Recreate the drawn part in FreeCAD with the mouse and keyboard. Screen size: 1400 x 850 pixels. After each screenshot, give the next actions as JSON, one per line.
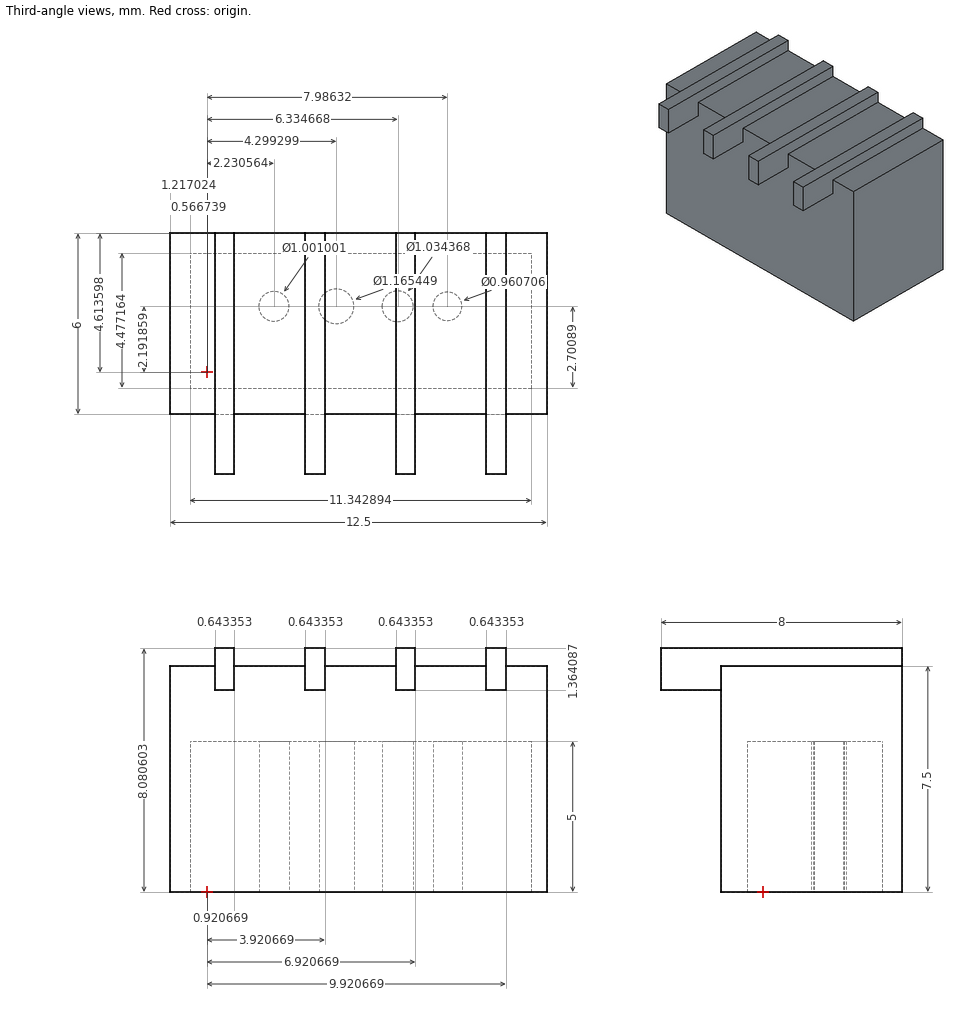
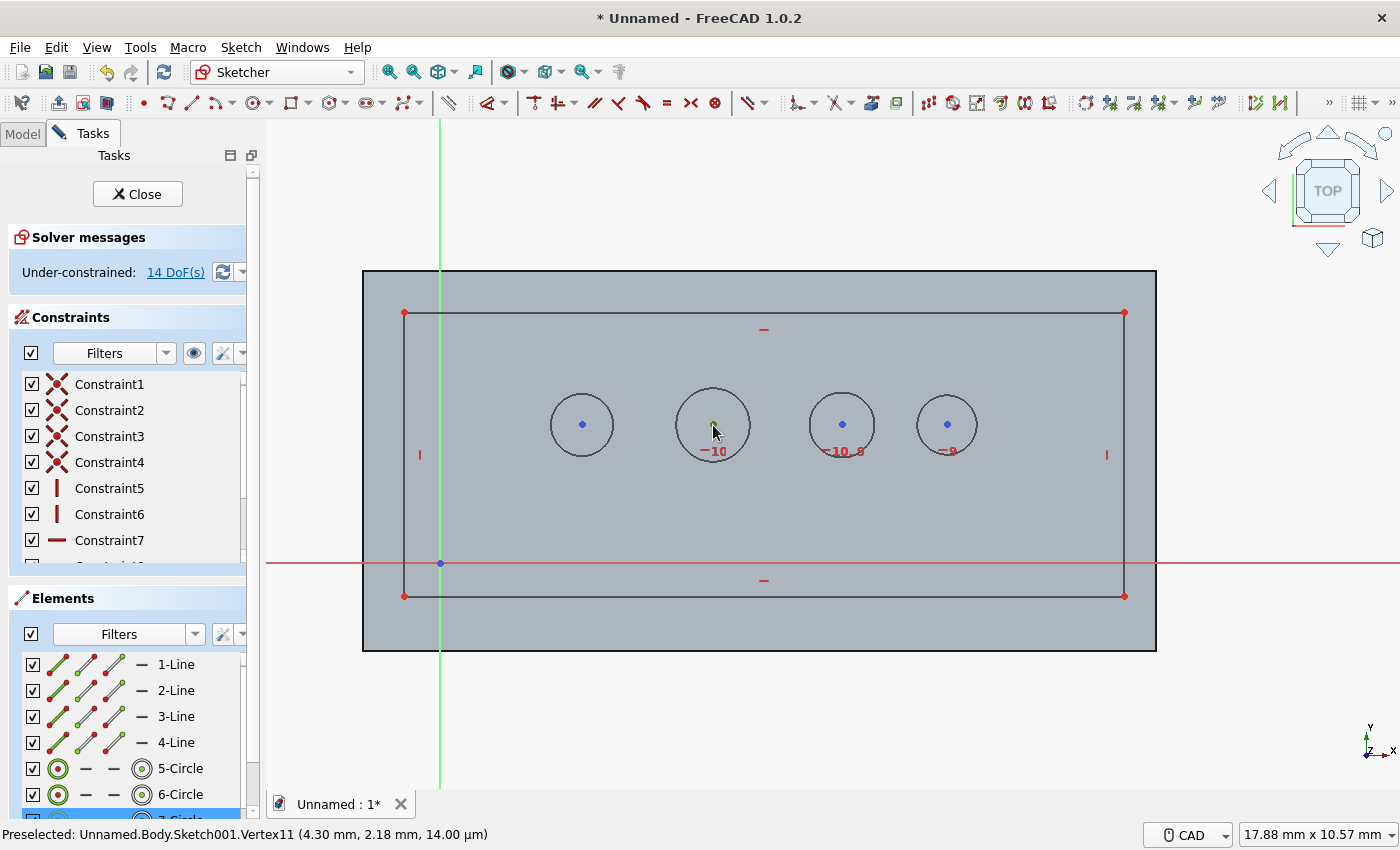
{"action": "left_click", "coordinate": [582, 425]}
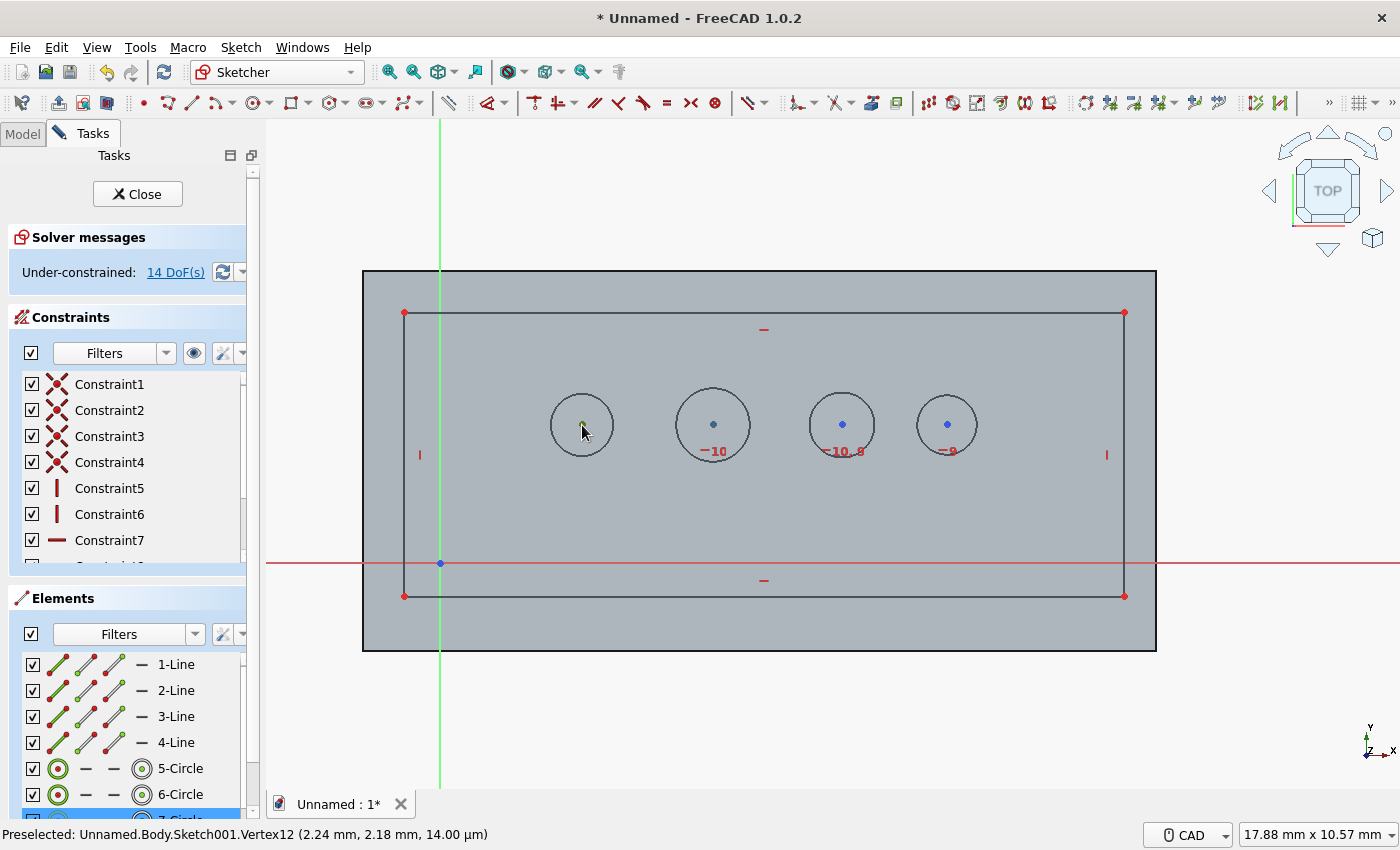
{"action": "key", "text": "h"}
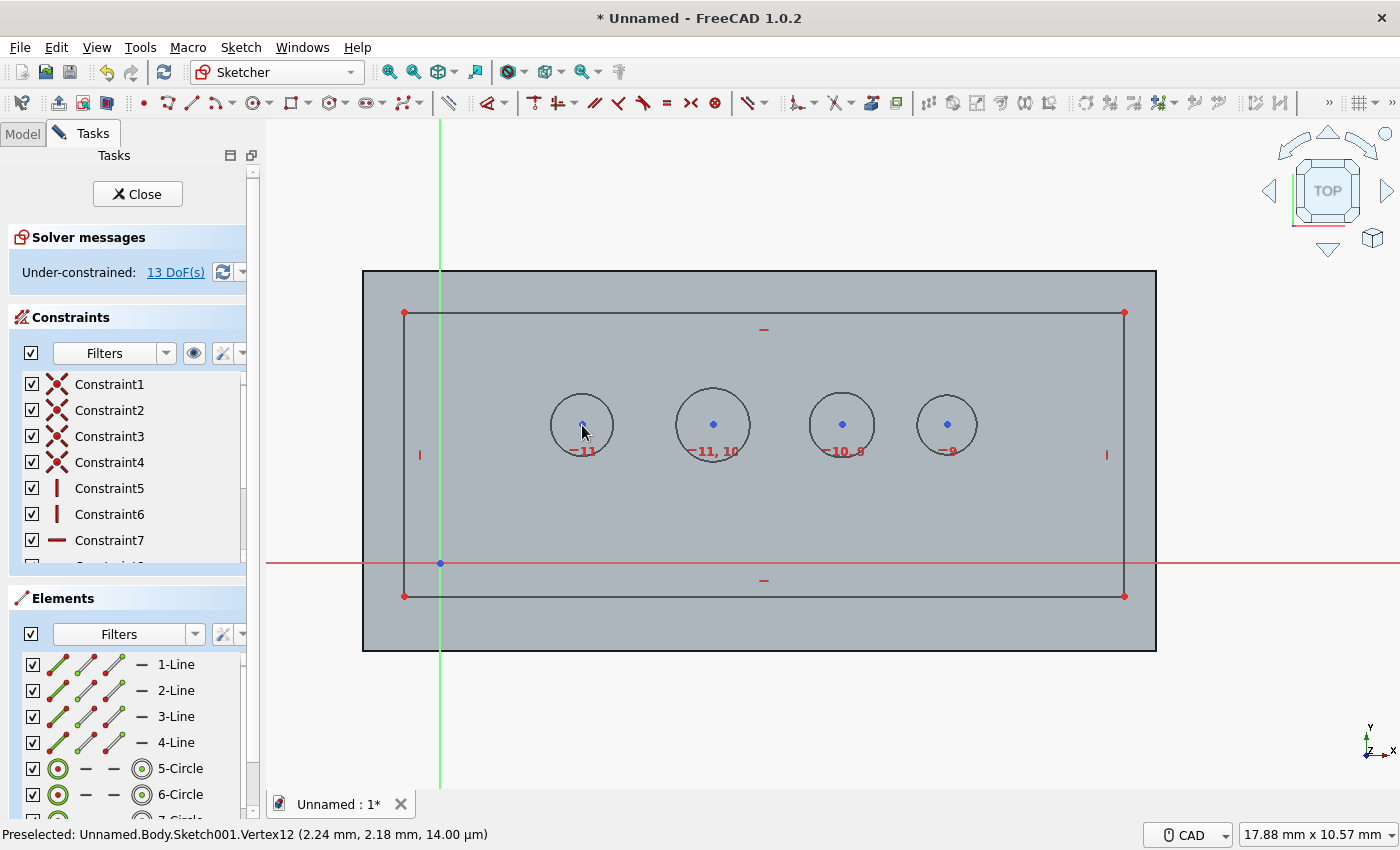
{"action": "key", "text": "d"}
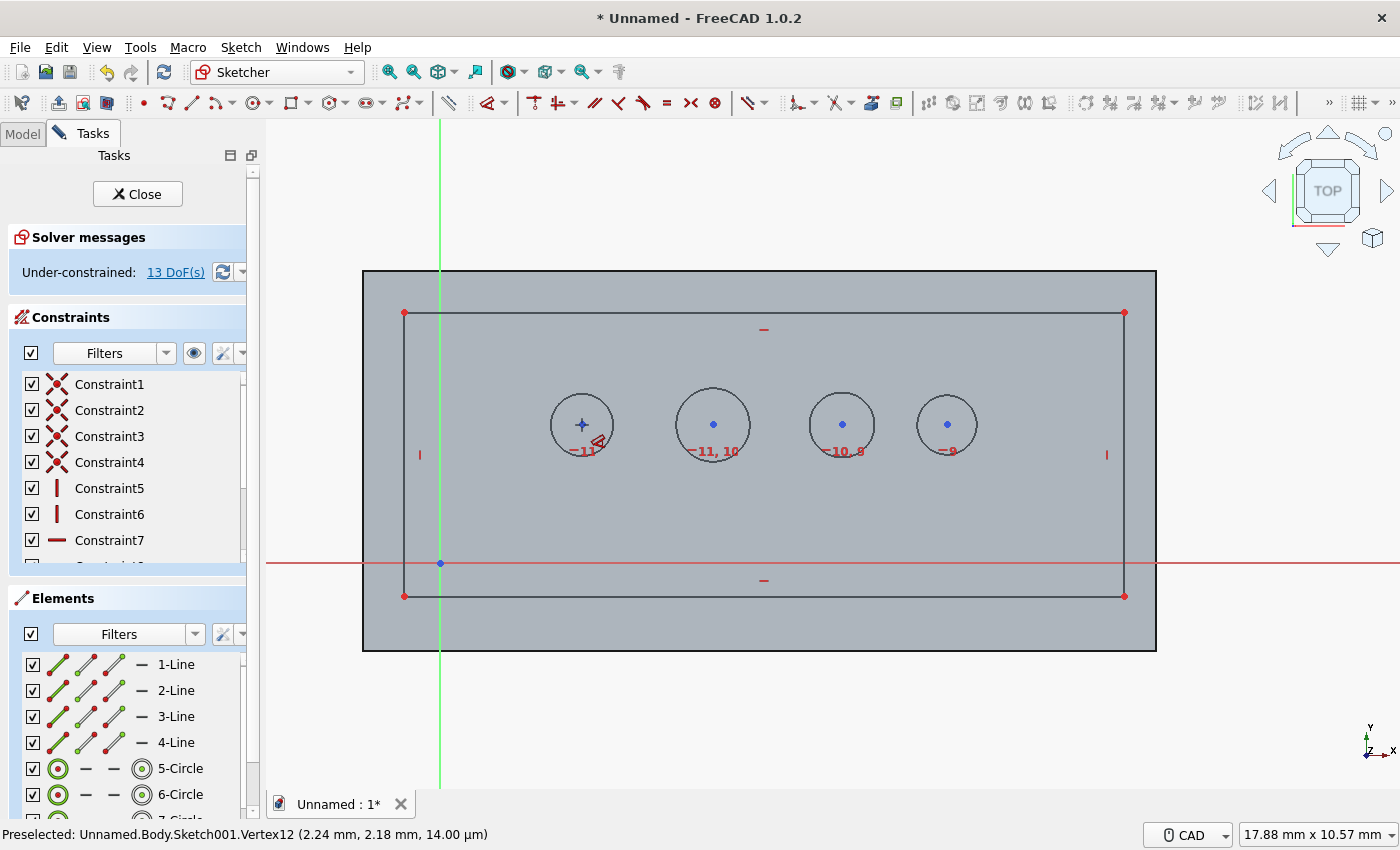
{"action": "left_click", "coordinate": [968, 404]}
{"action": "left_click", "coordinate": [991, 381]}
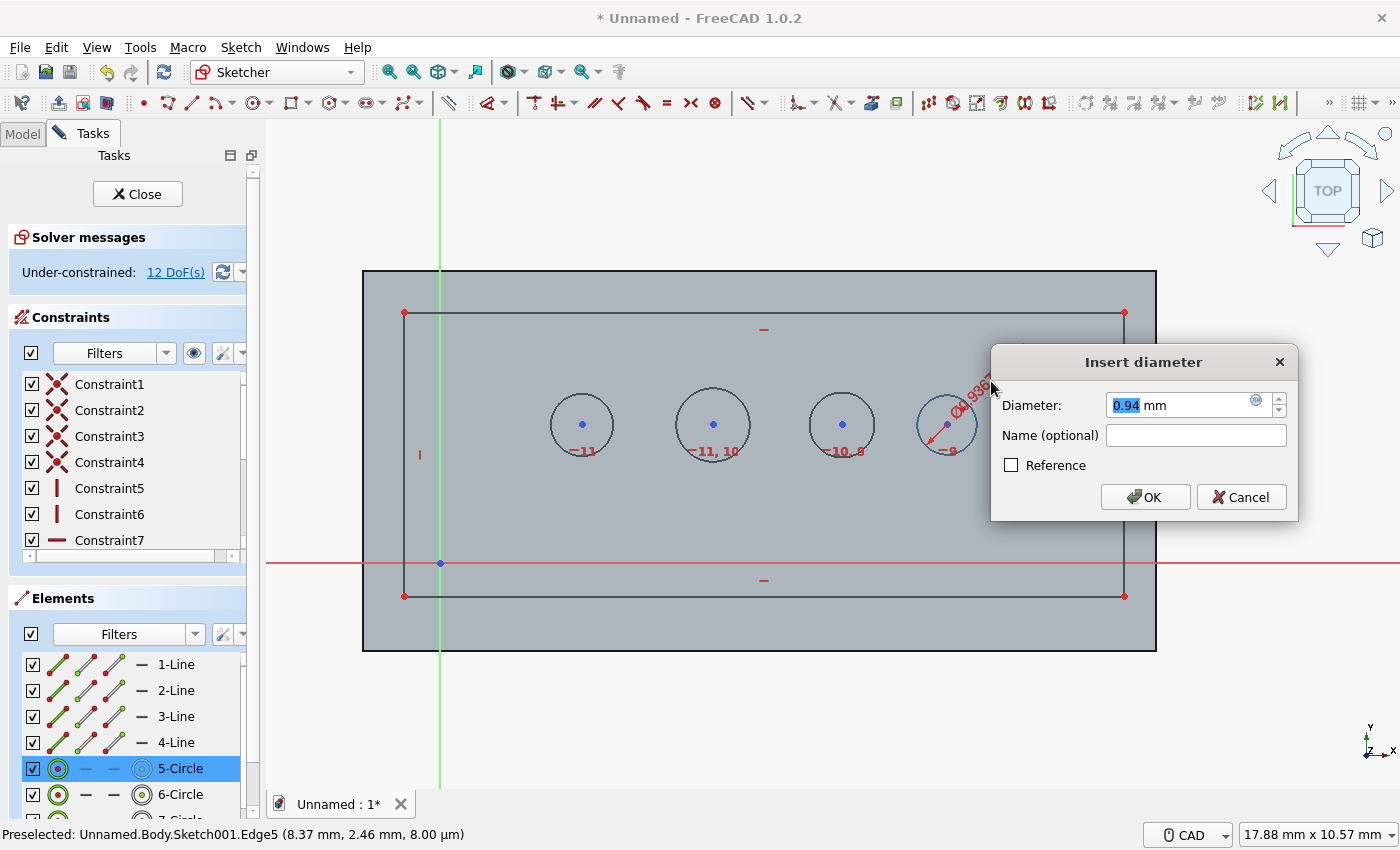
{"action": "type", "text": "0.960706"}
{"action": "key", "text": "Return"}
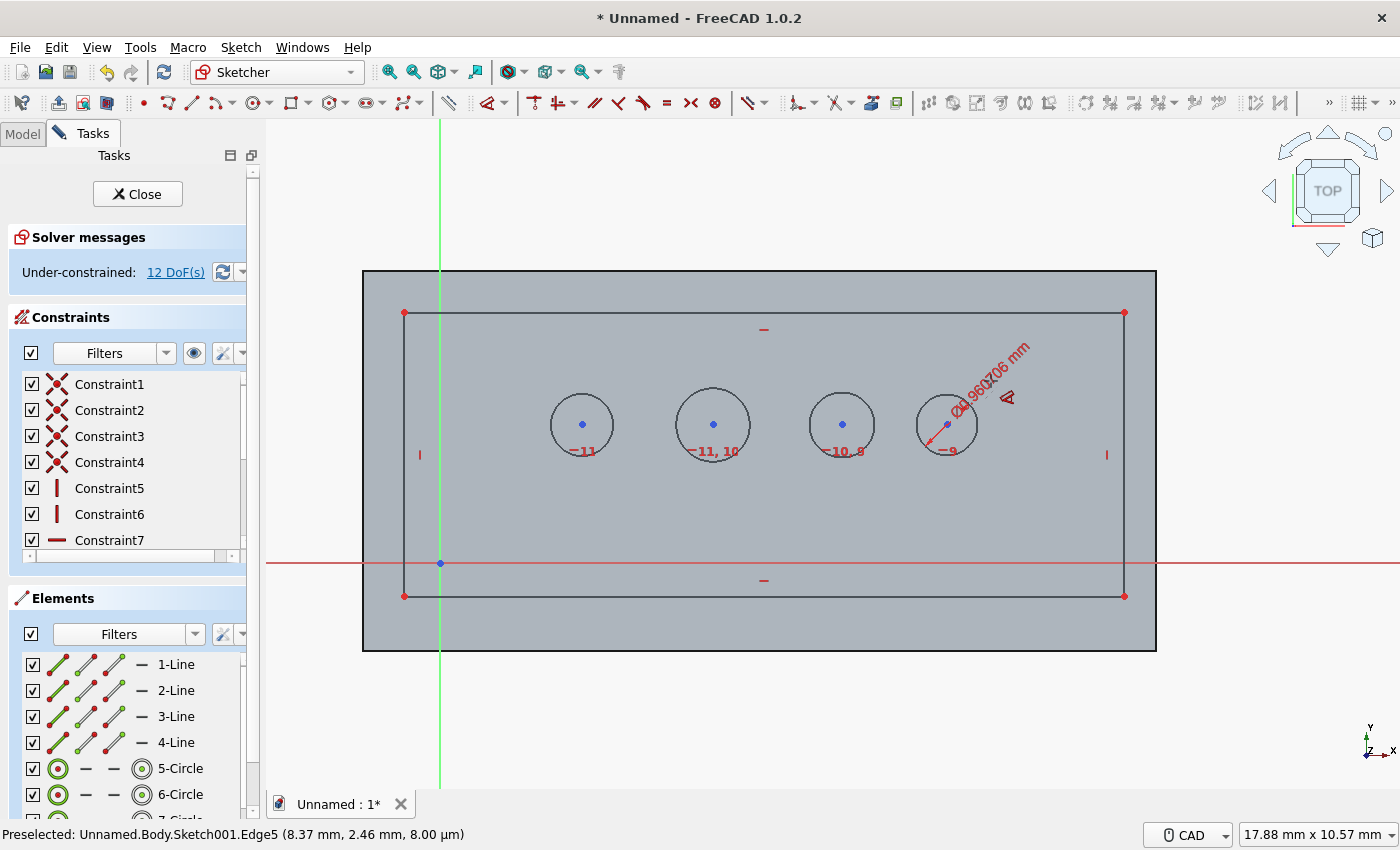
{"action": "left_click", "coordinate": [865, 402]}
{"action": "left_click", "coordinate": [888, 379]}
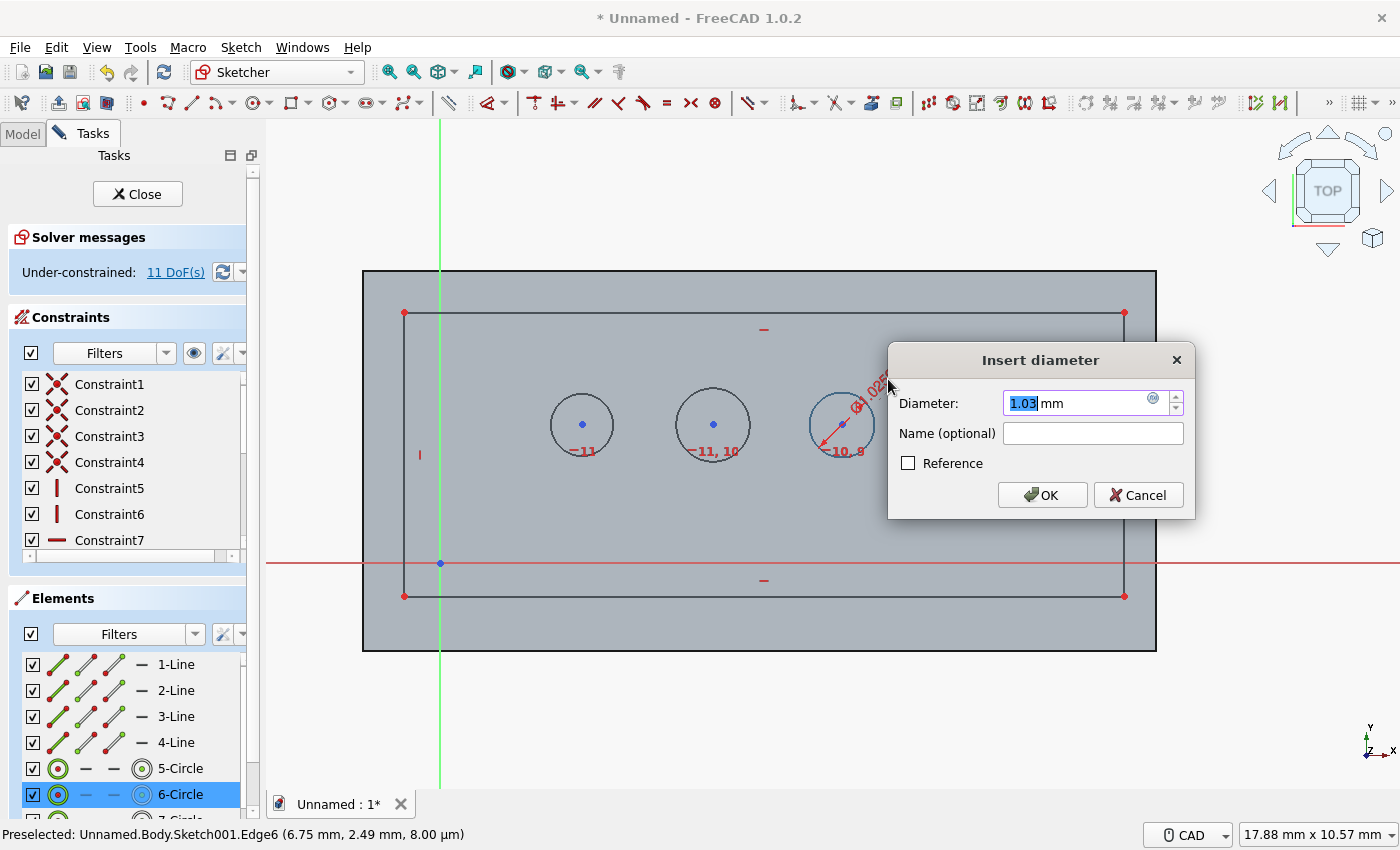
{"action": "type", "text": "1.034368"}
{"action": "key", "text": "Return"}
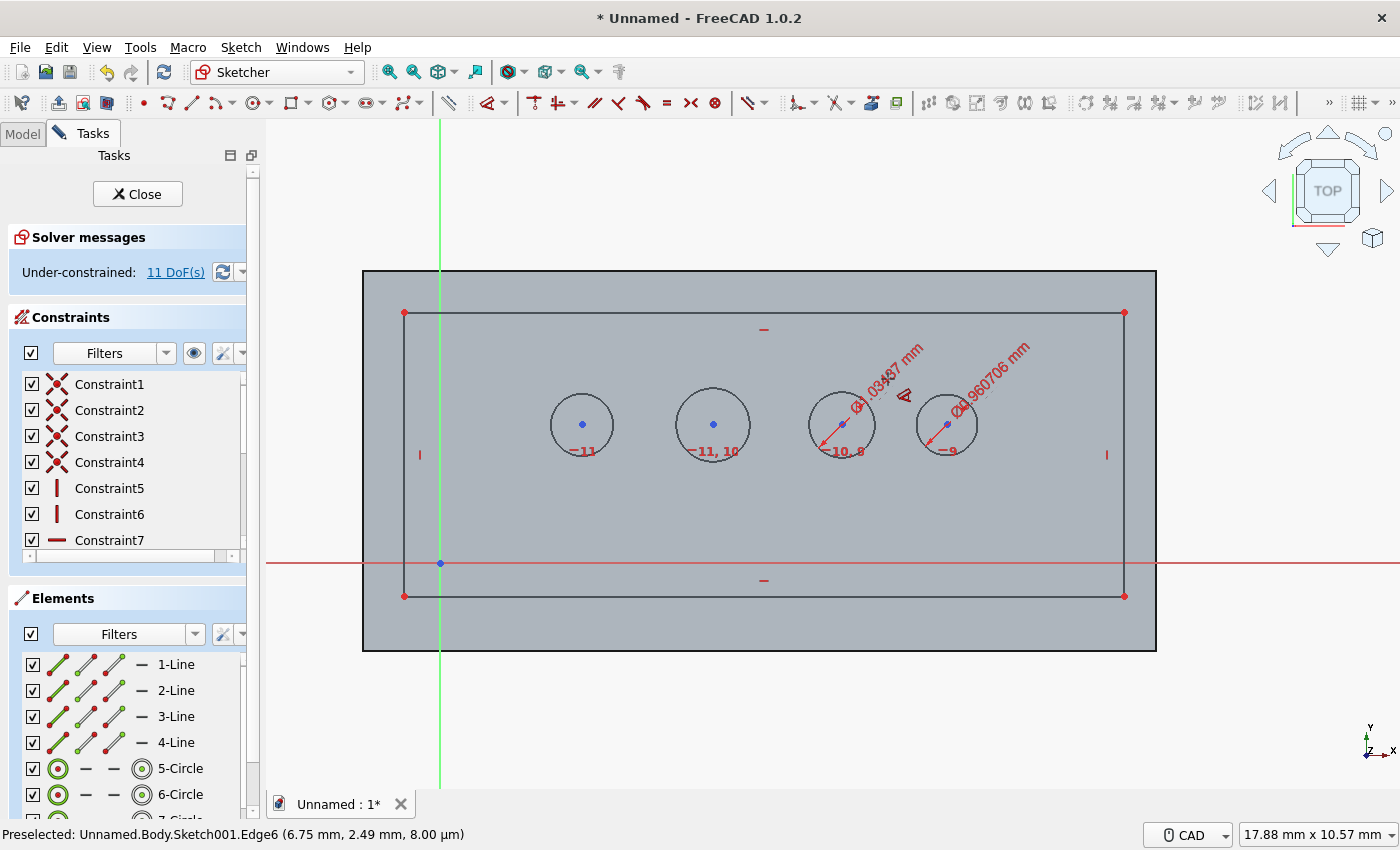
{"action": "left_click", "coordinate": [739, 399]}
{"action": "left_click", "coordinate": [762, 376]}